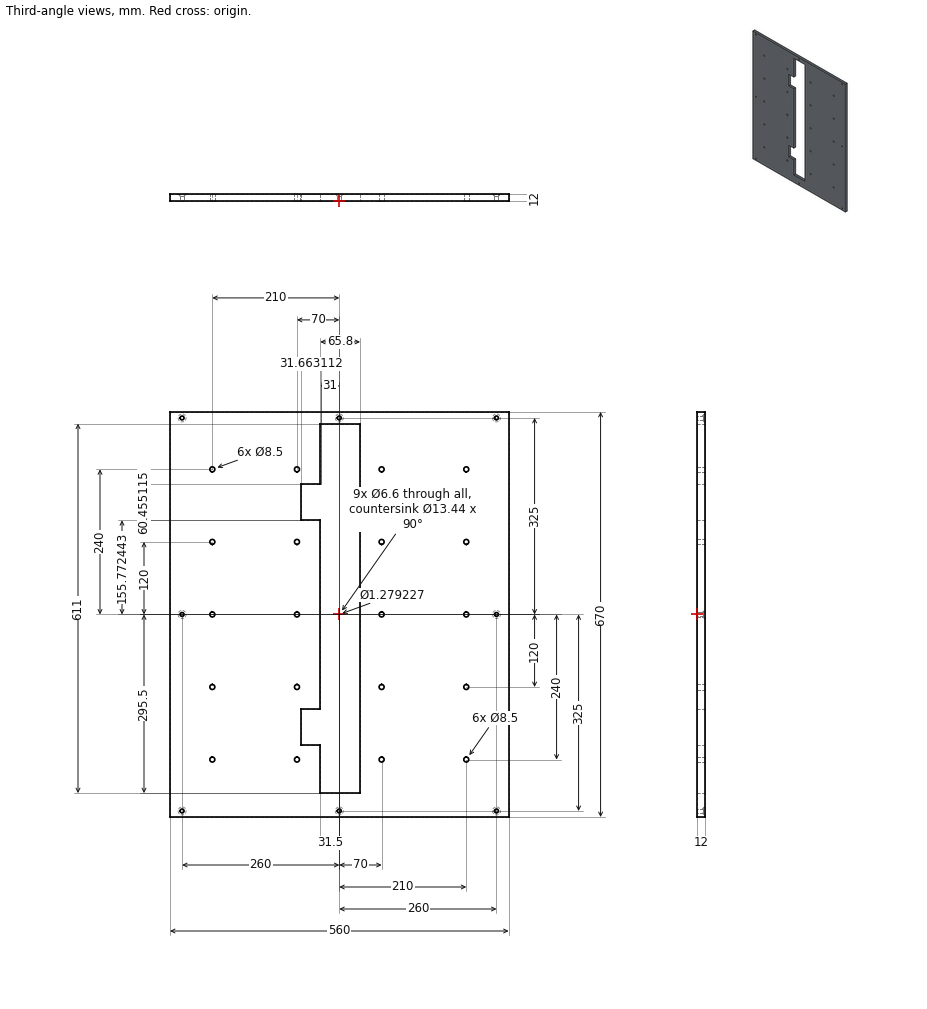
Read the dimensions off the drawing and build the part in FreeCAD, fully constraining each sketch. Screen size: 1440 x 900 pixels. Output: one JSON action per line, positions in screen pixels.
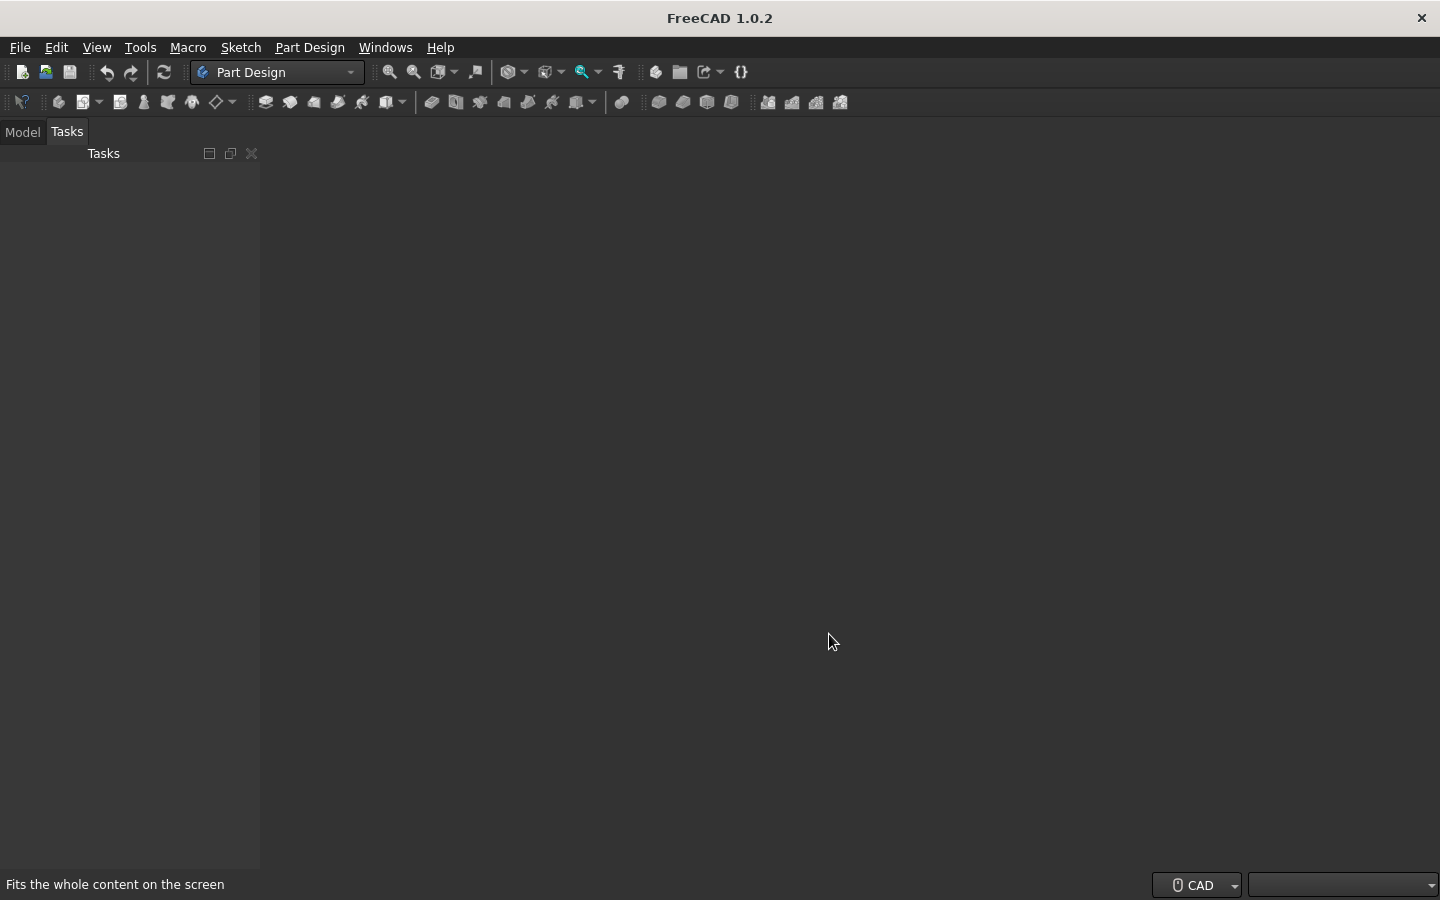
{"action": "left_click", "coordinate": [22, 72]}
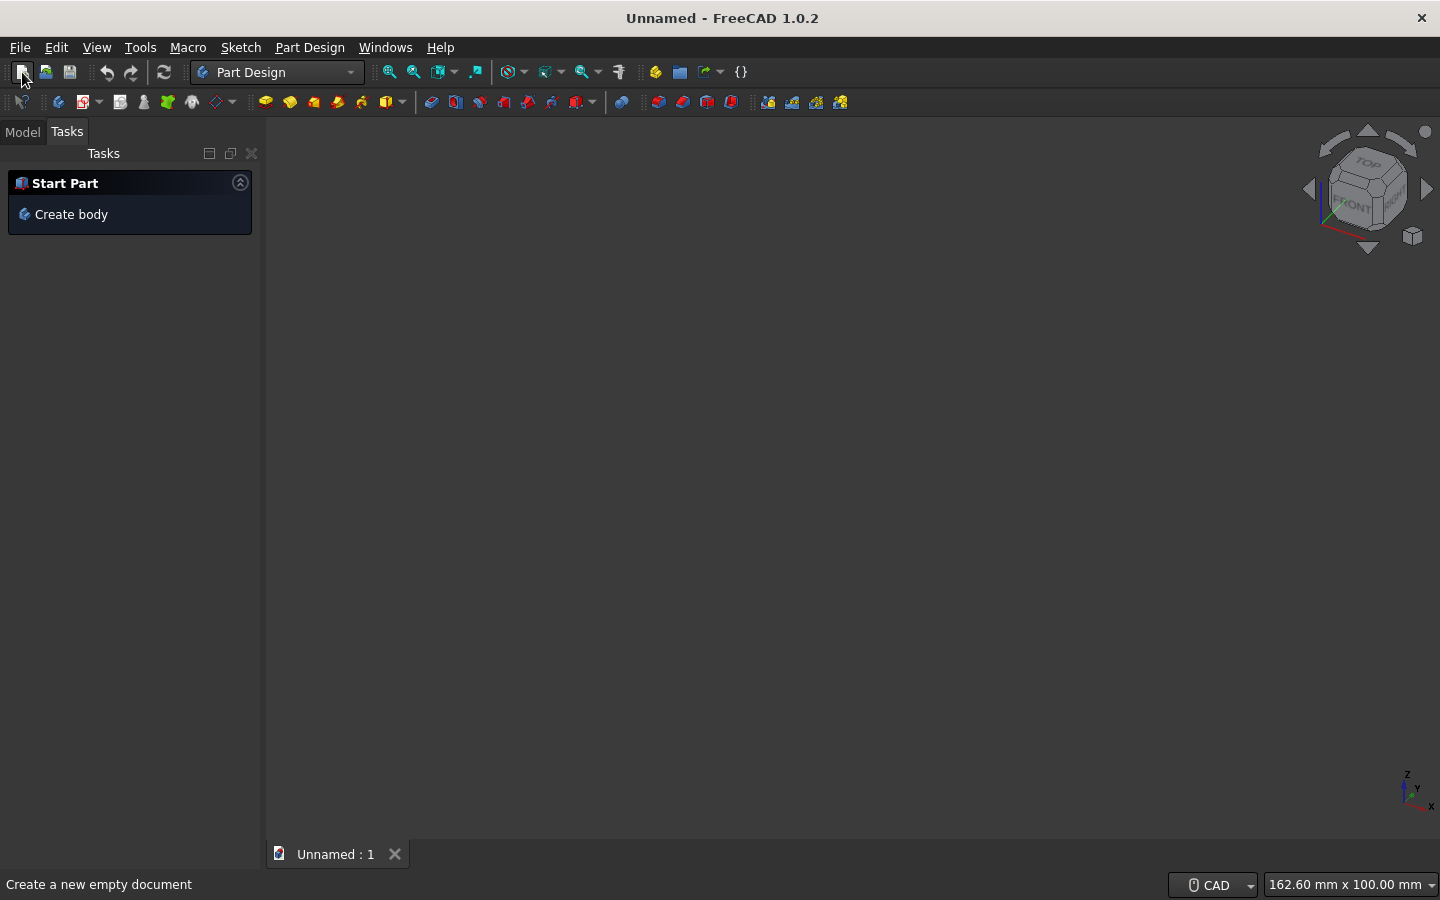
{"action": "left_click", "coordinate": [84, 102]}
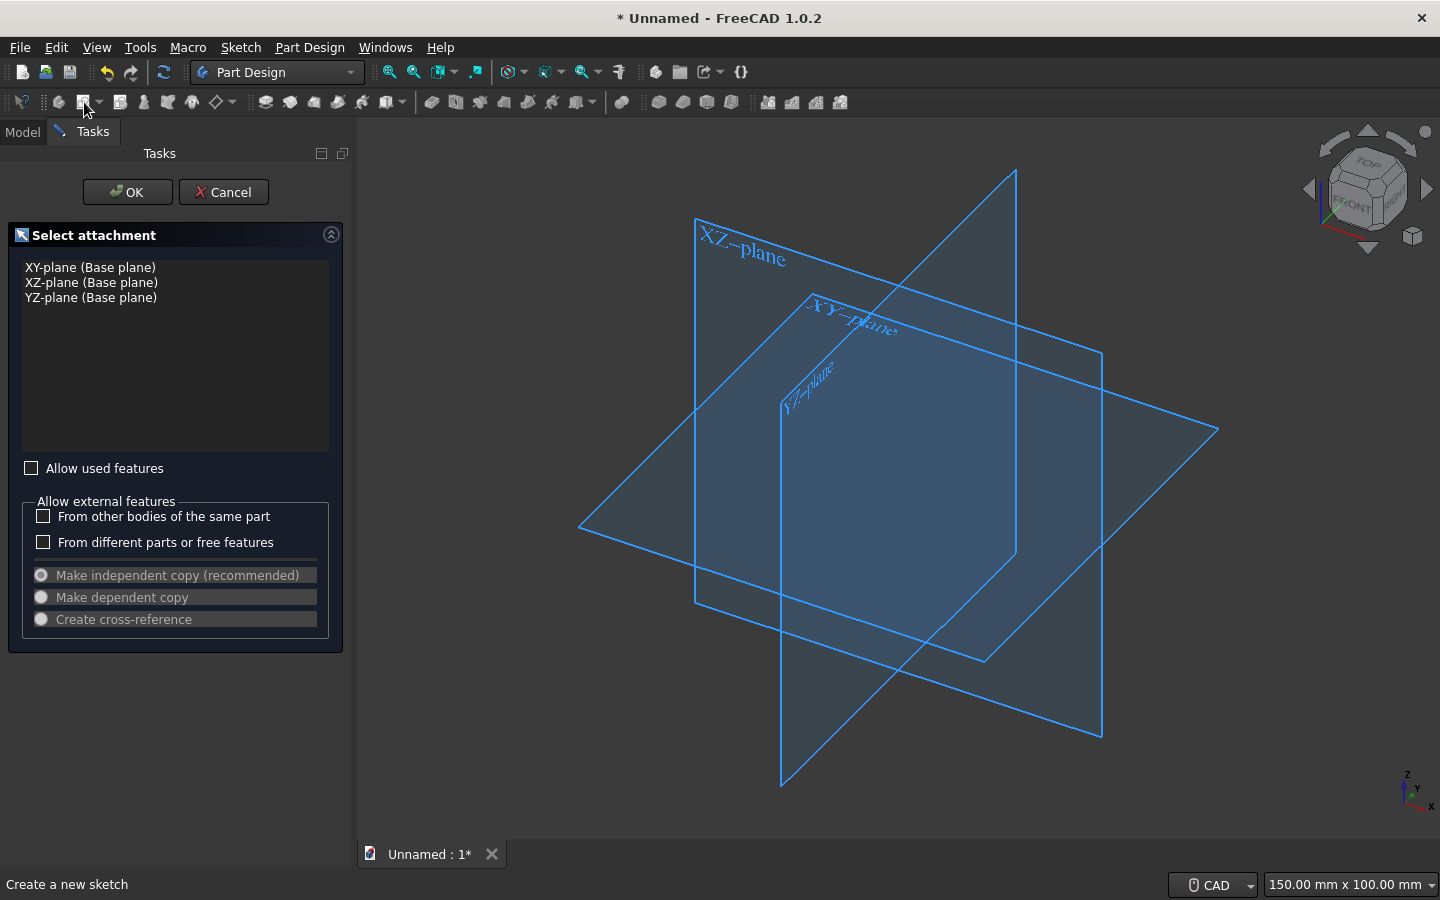
{"action": "left_click", "coordinate": [82, 282]}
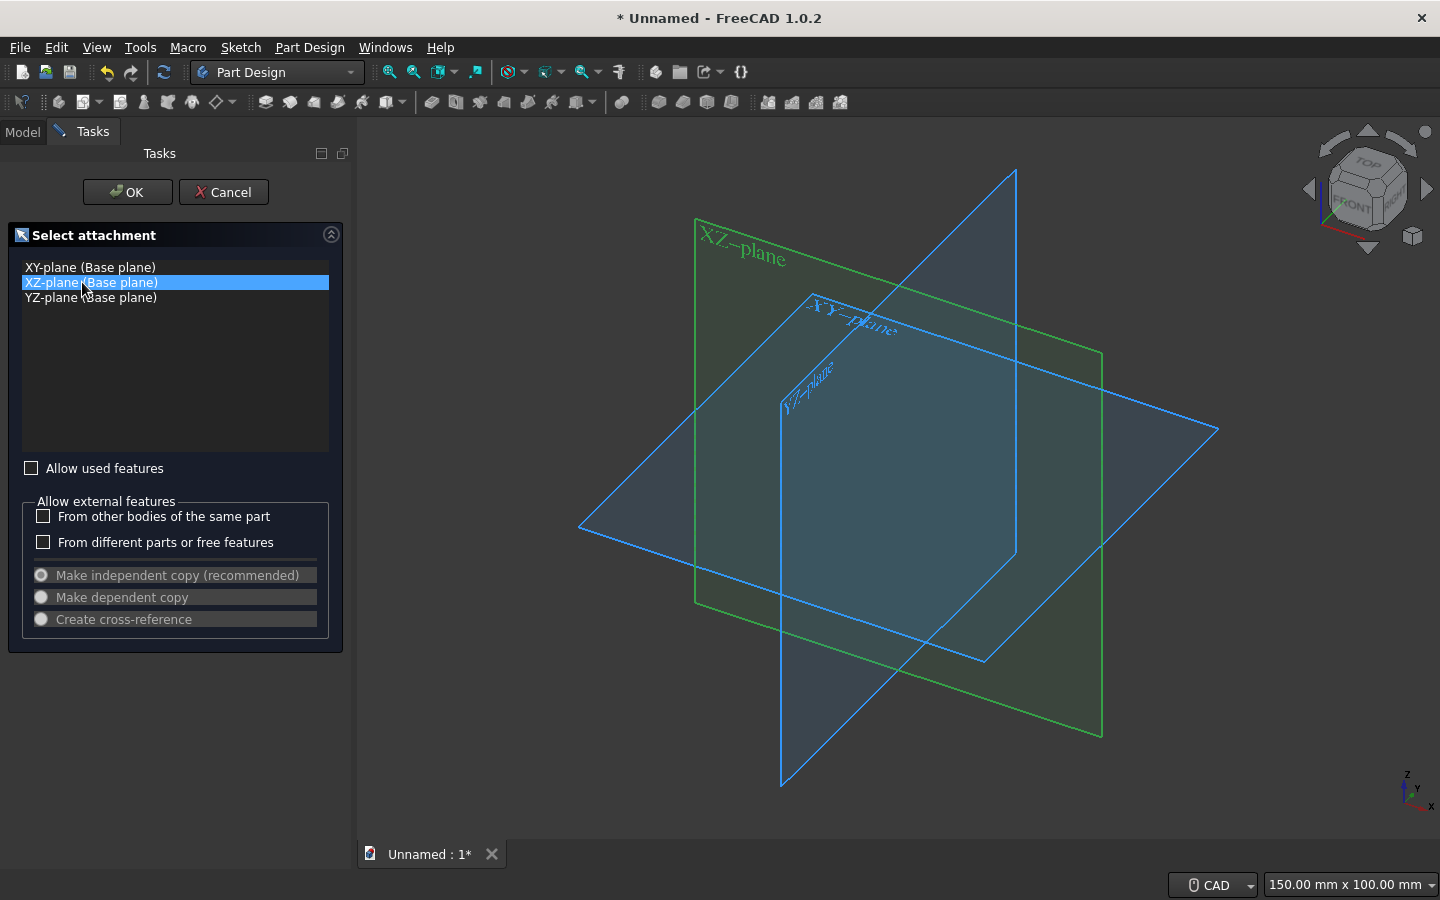
{"action": "left_click", "coordinate": [128, 192]}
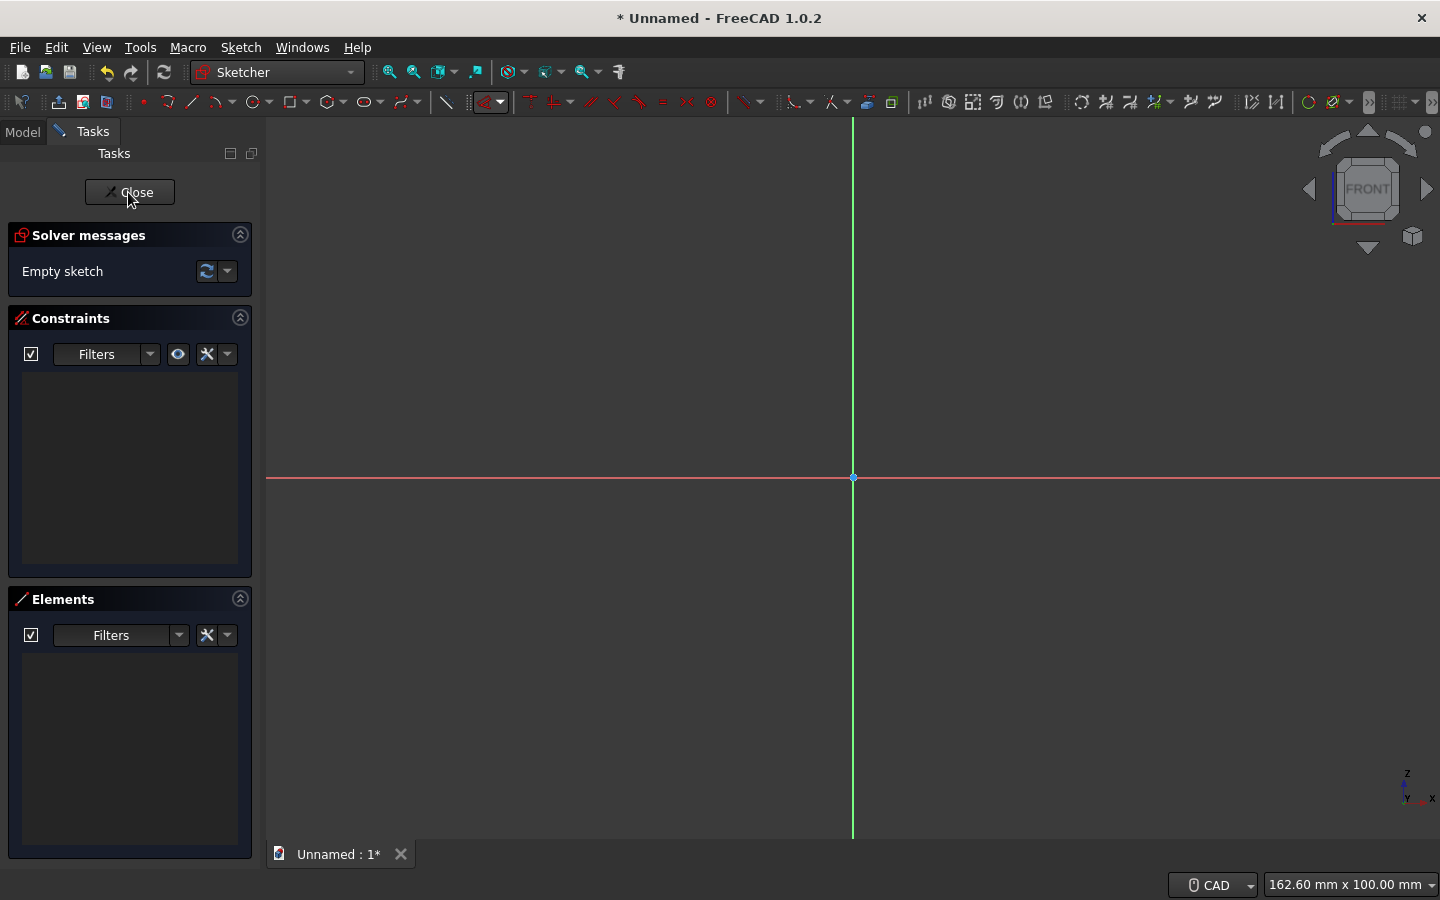
{"action": "scroll", "coordinate": [778, 478], "scroll_direction": "down", "scroll_amount": 12}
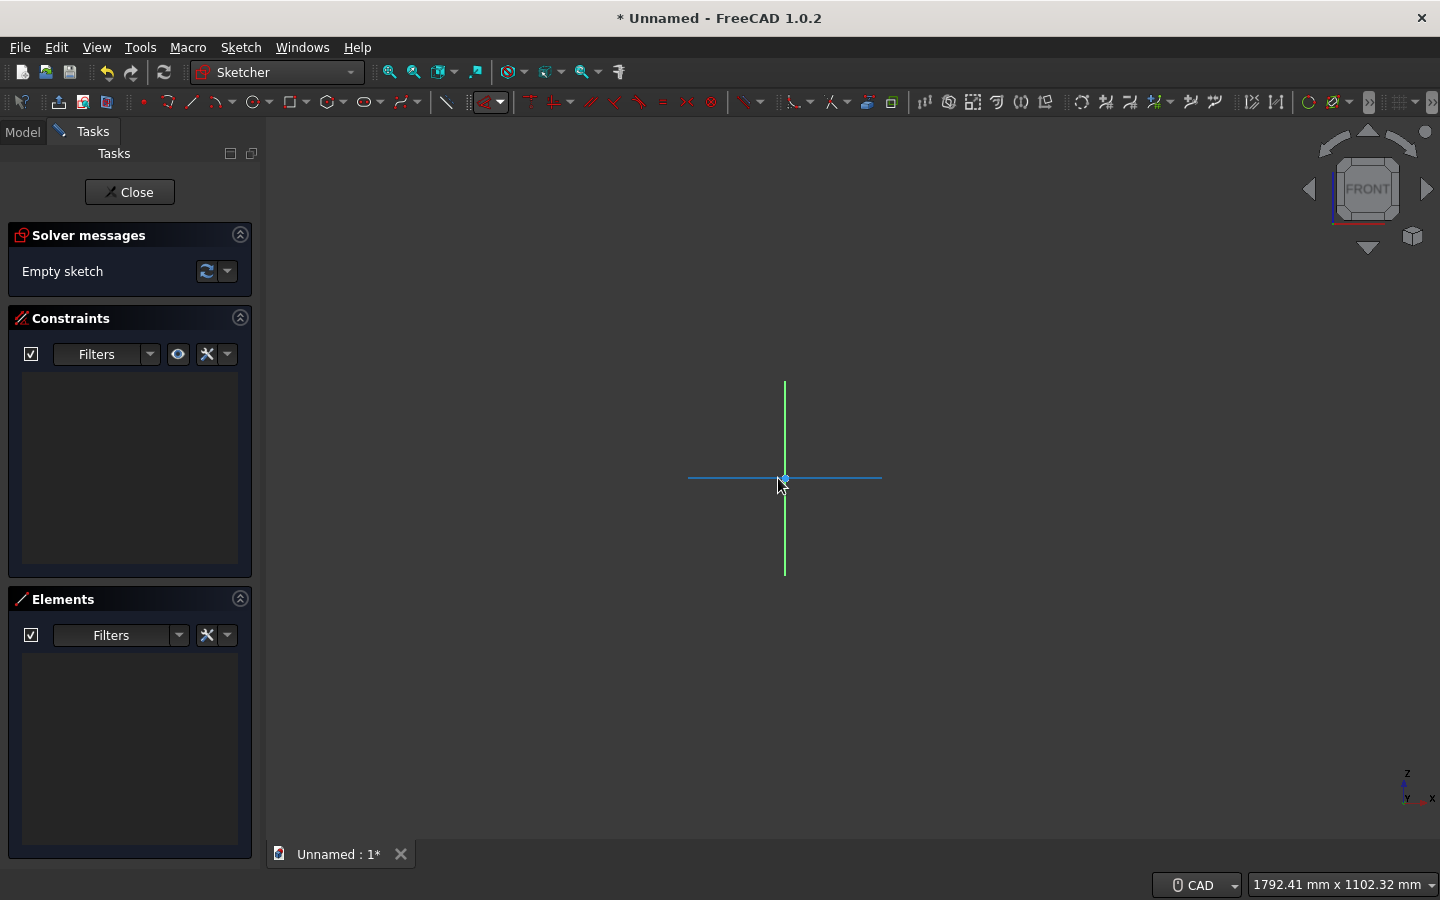
{"action": "left_click", "coordinate": [308, 102]}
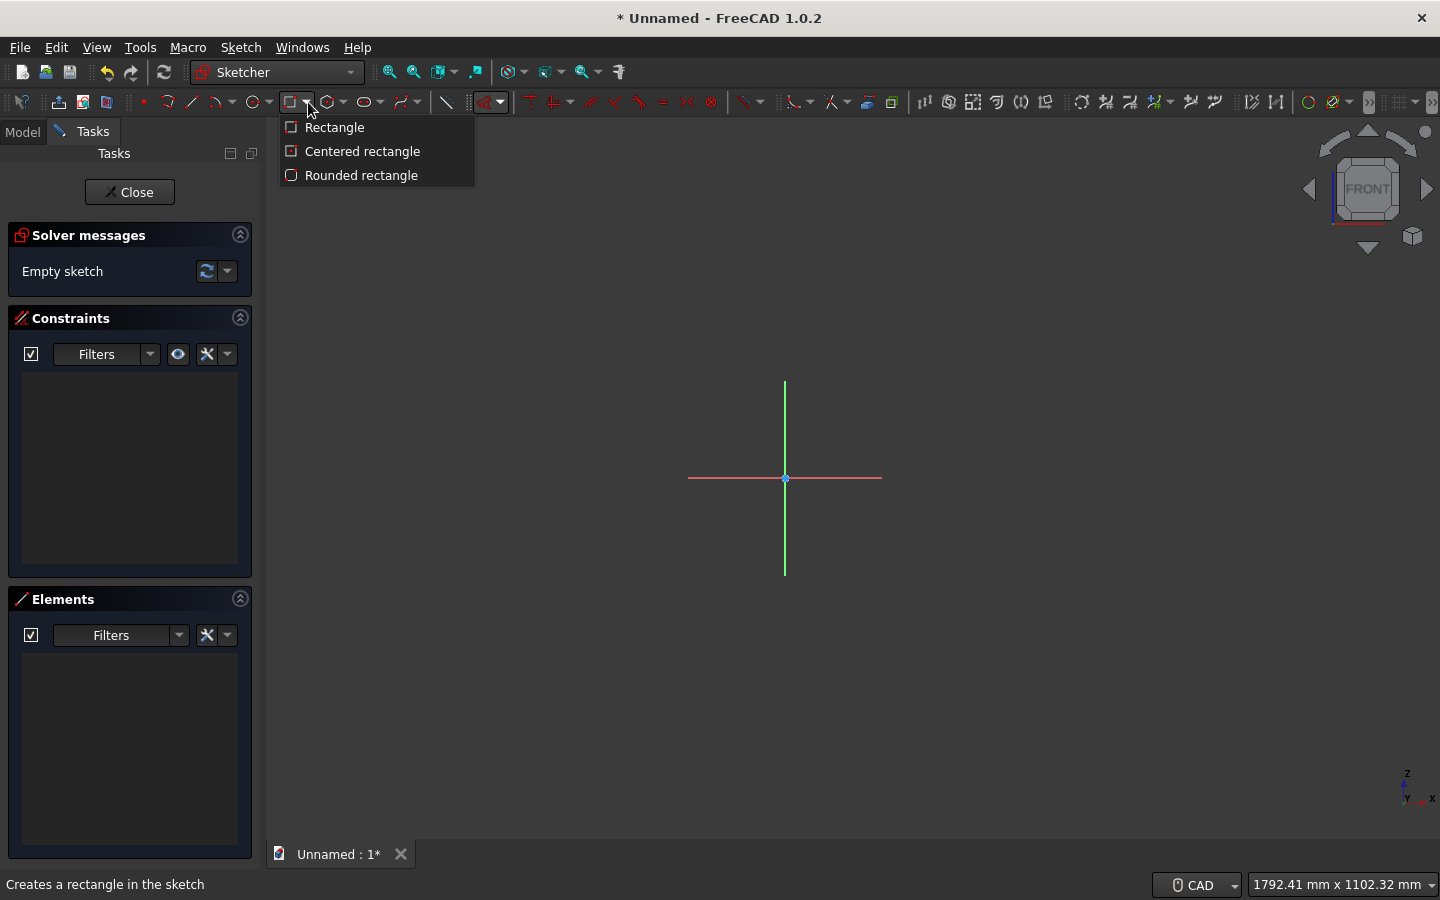
{"action": "left_click", "coordinate": [378, 151]}